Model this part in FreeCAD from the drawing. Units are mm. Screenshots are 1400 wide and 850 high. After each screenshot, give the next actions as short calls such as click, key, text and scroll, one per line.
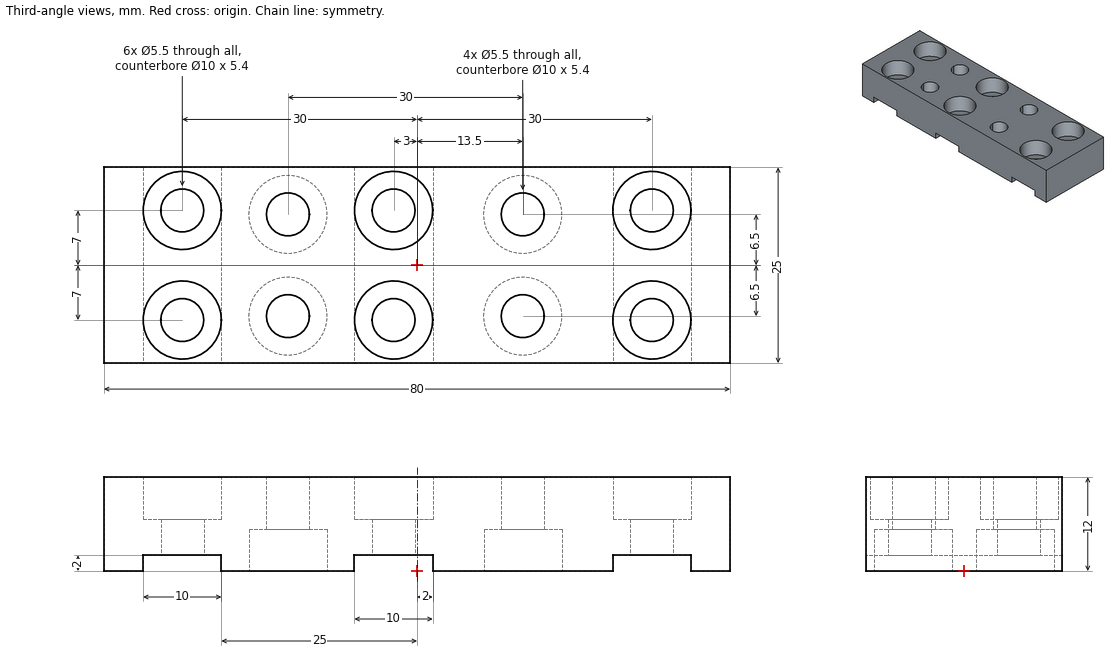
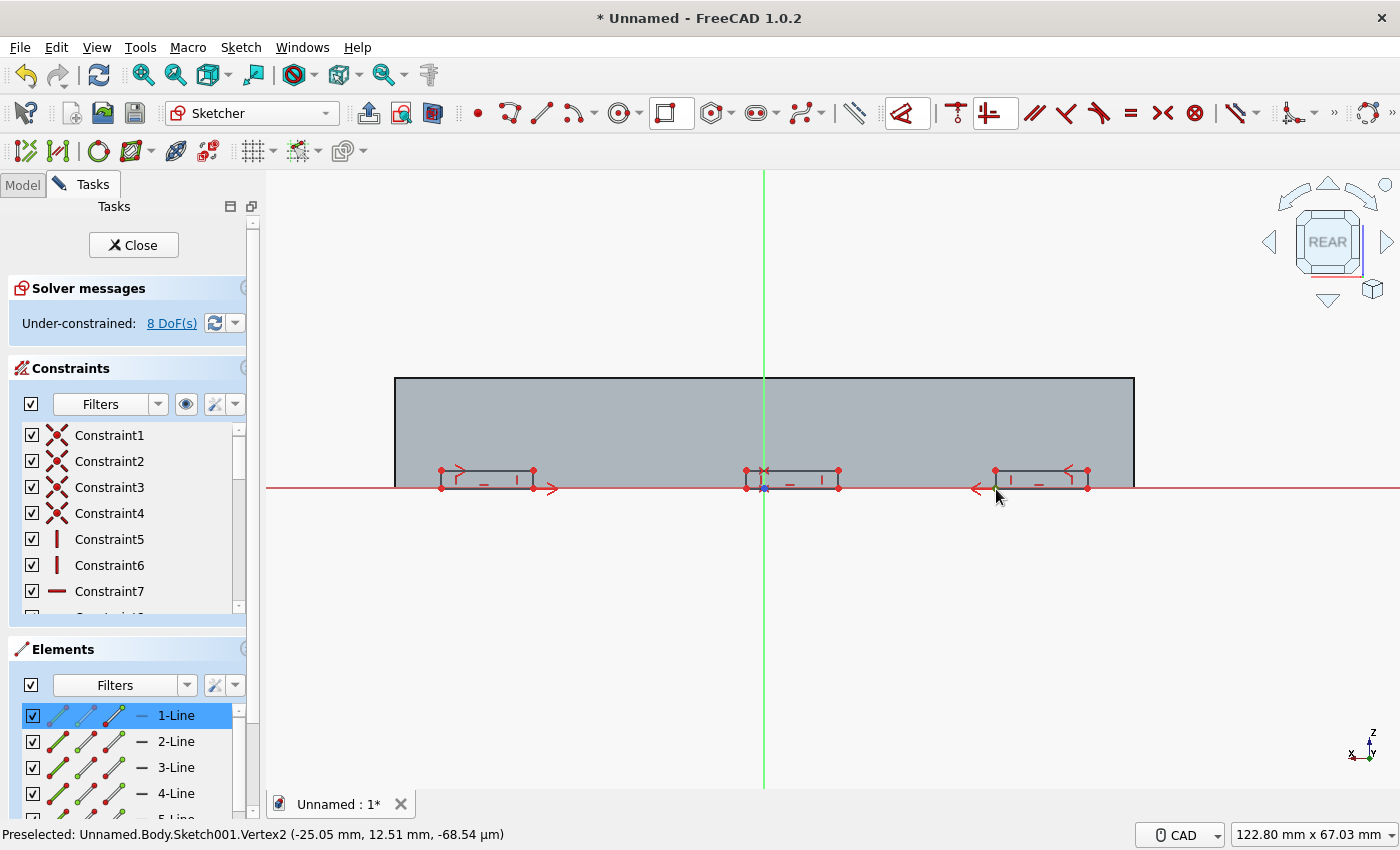
click(361, 488)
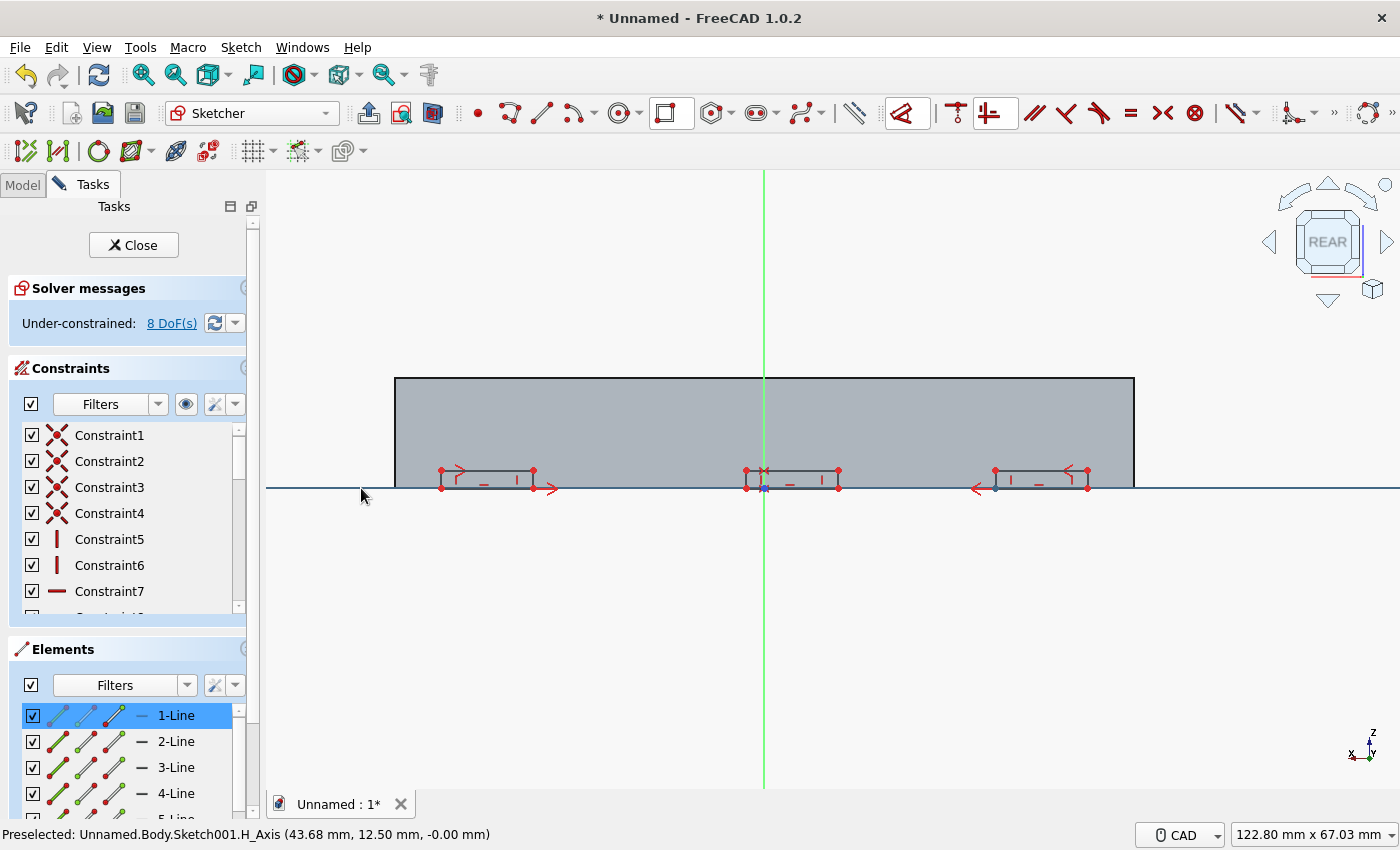
click(956, 114)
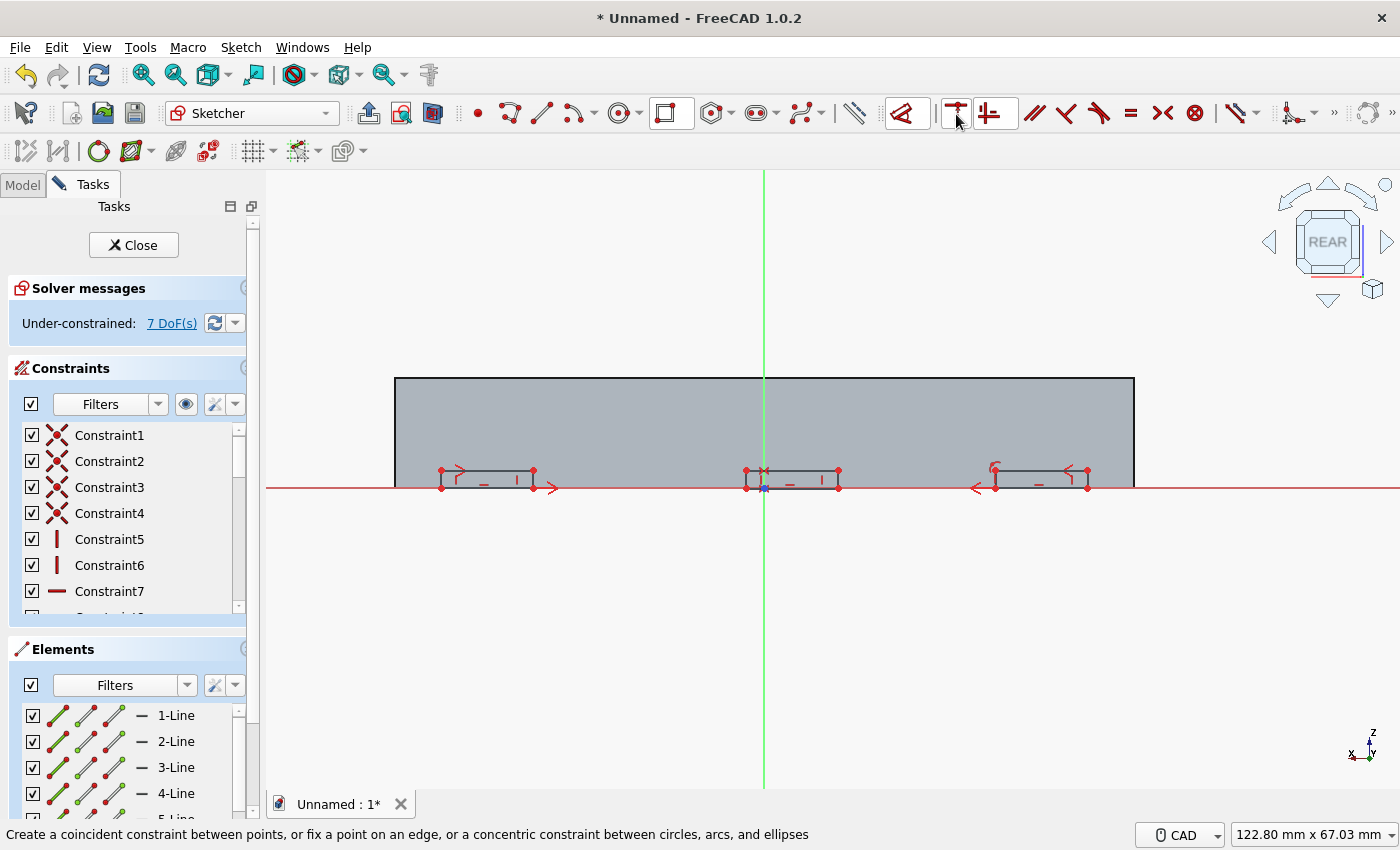
click(746, 489)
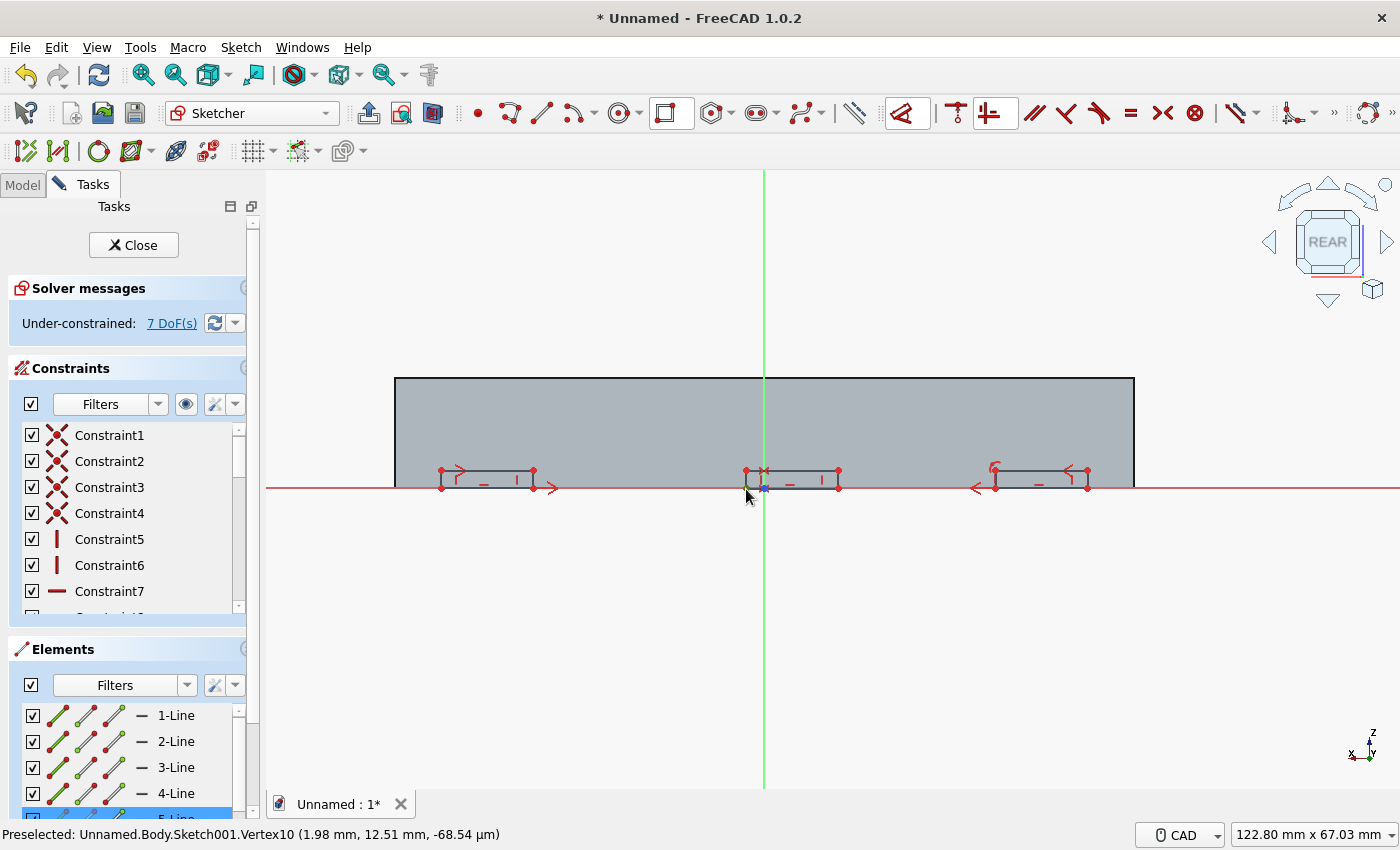
click(361, 488)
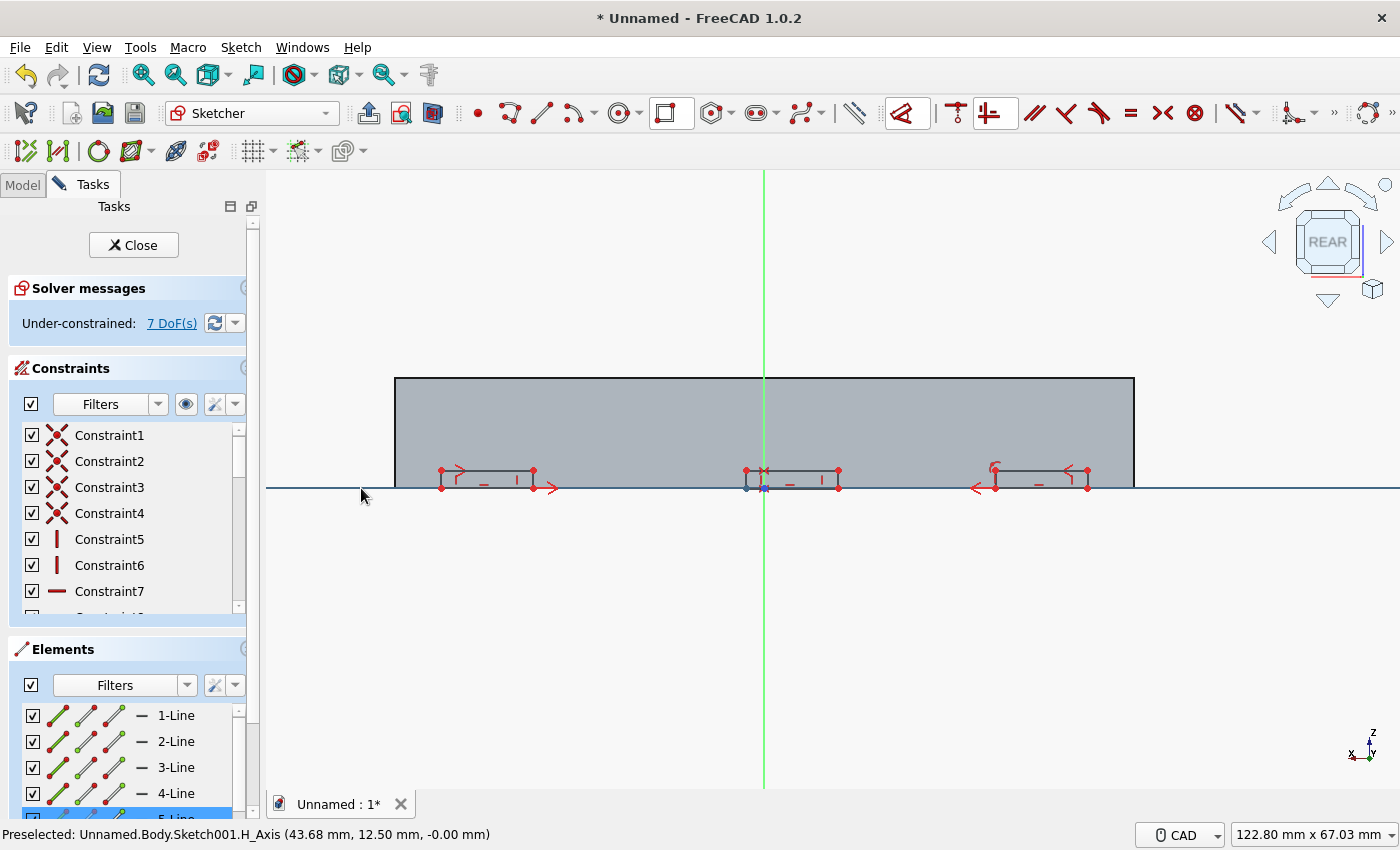
click(956, 114)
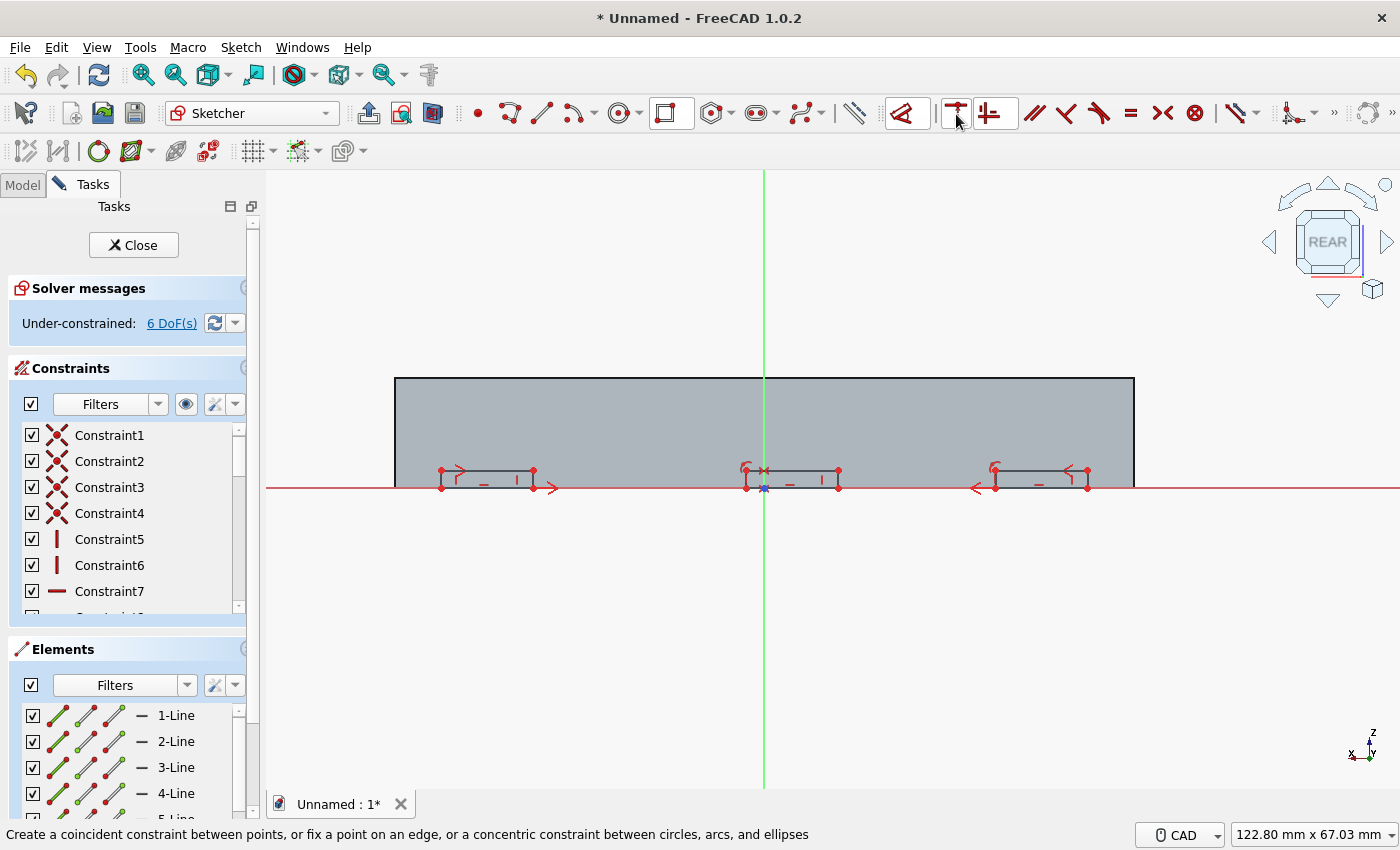
scroll(996, 480, up, 4)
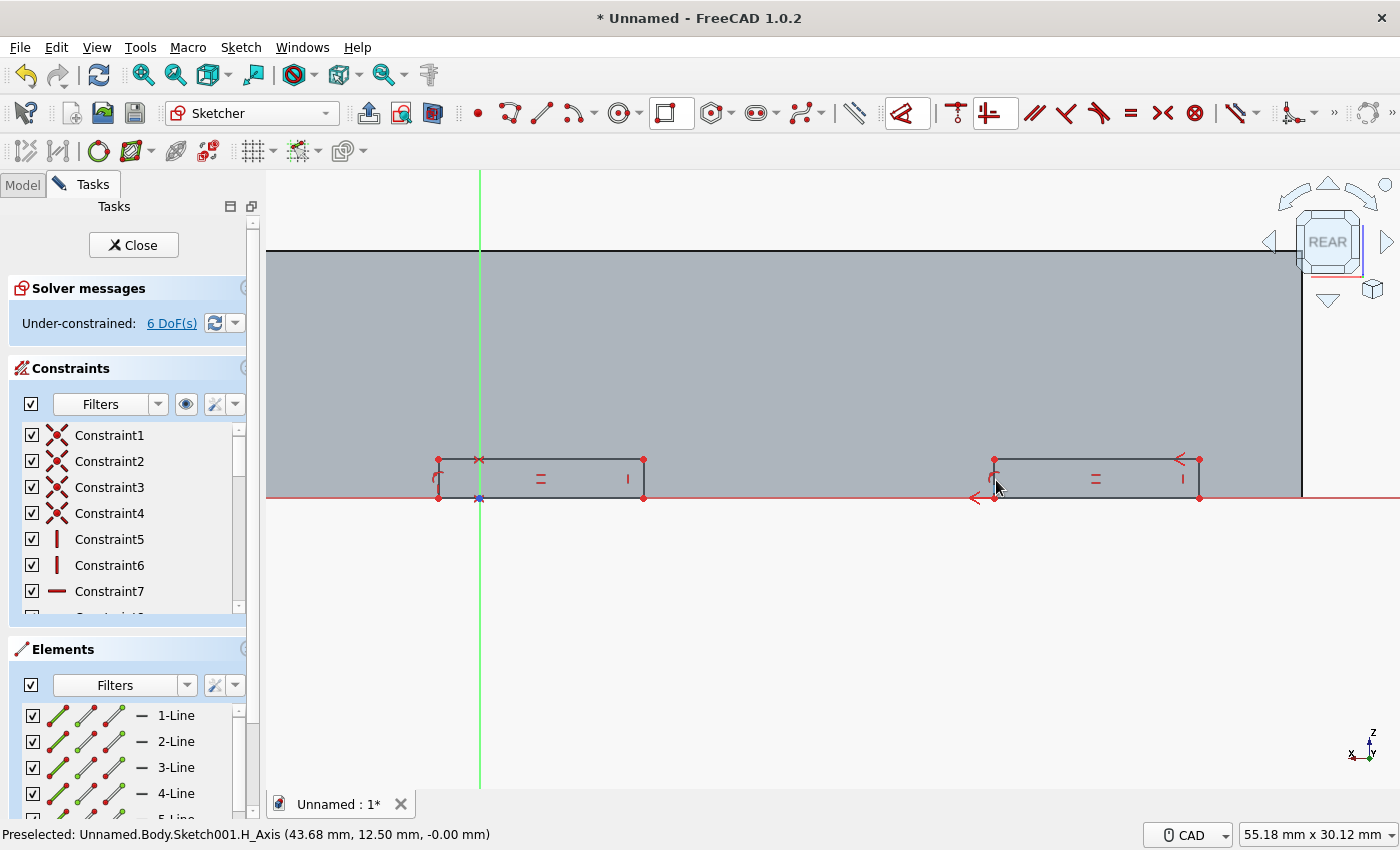
click(994, 467)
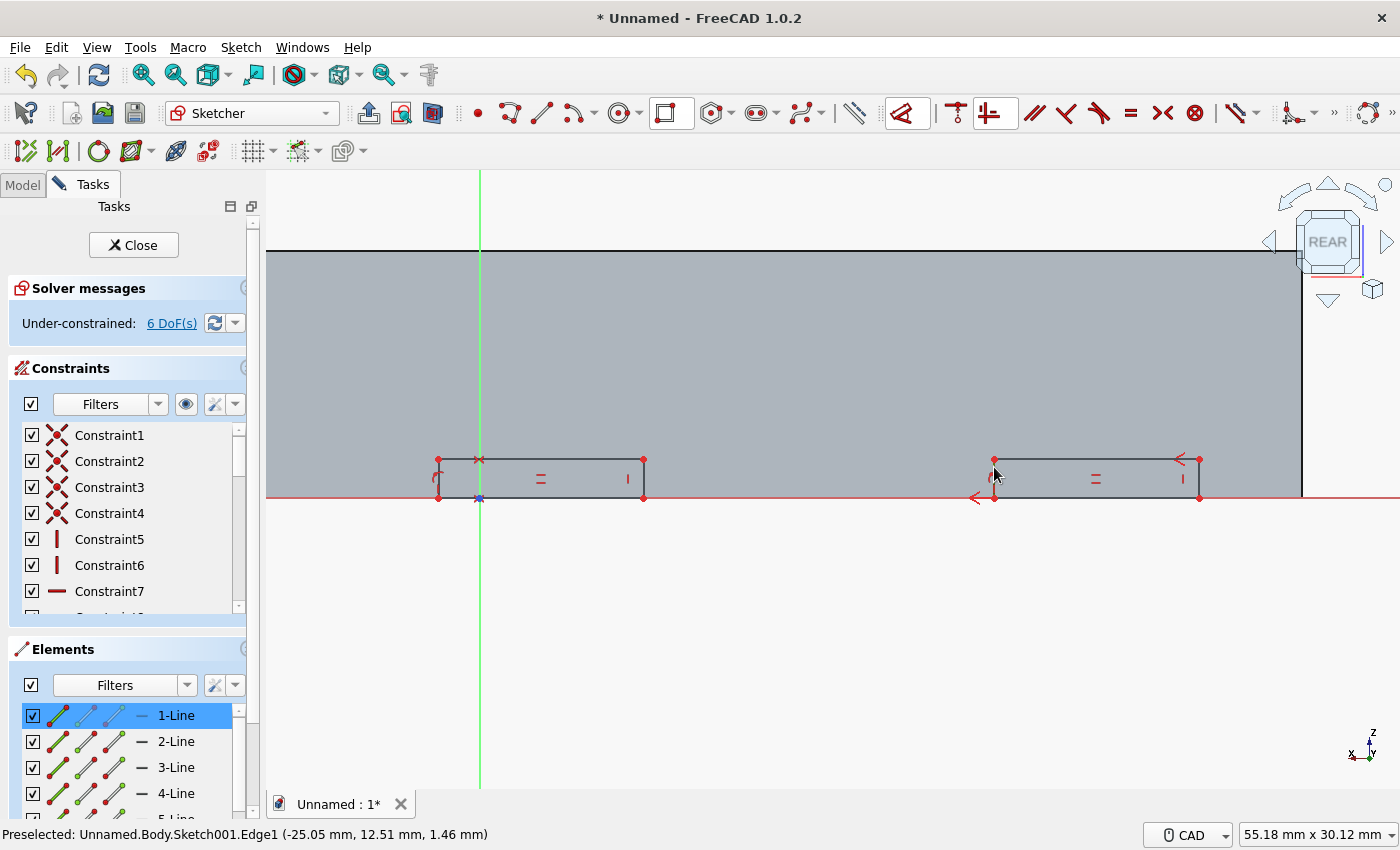
key(i)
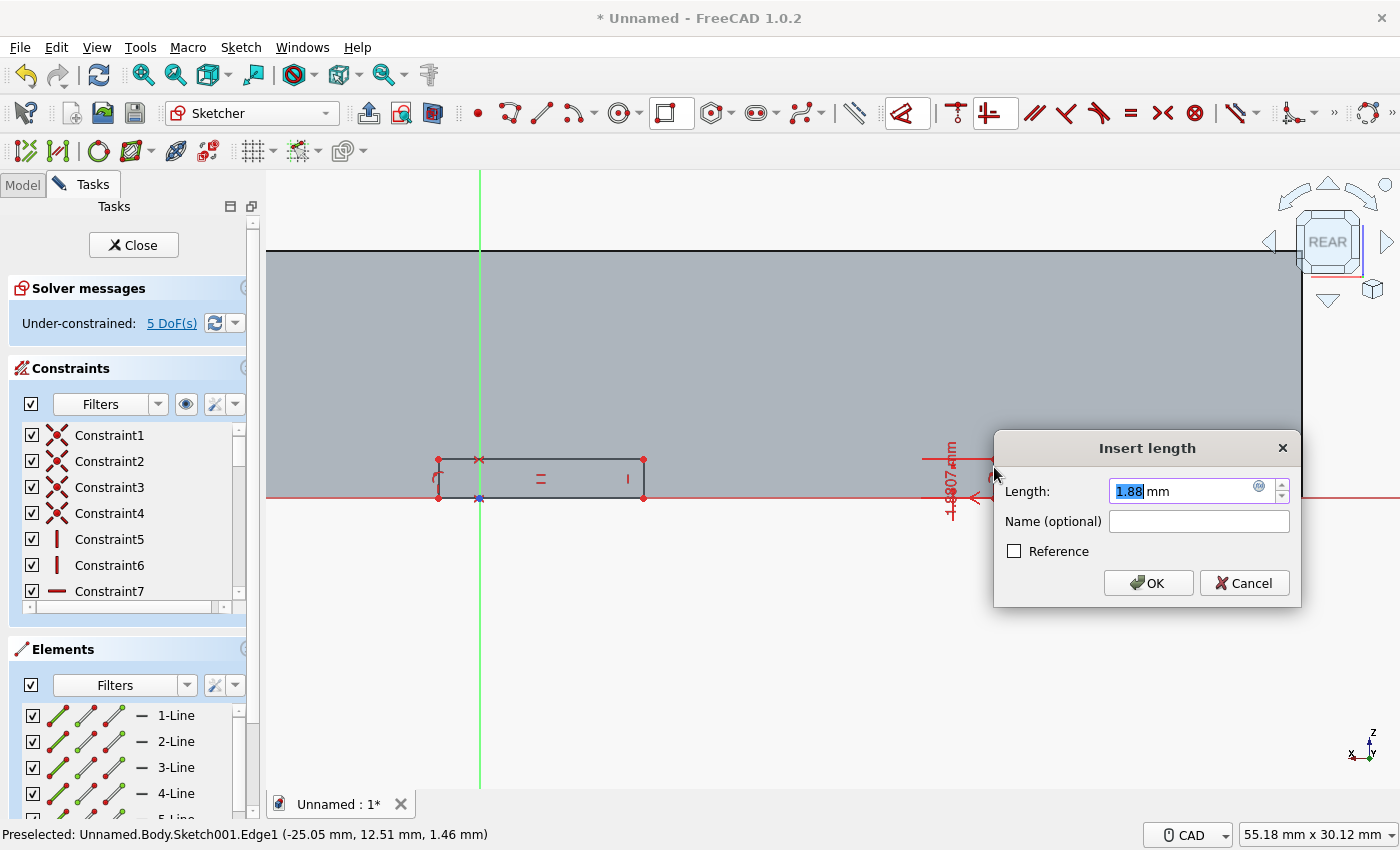
text(2)
key(Return)